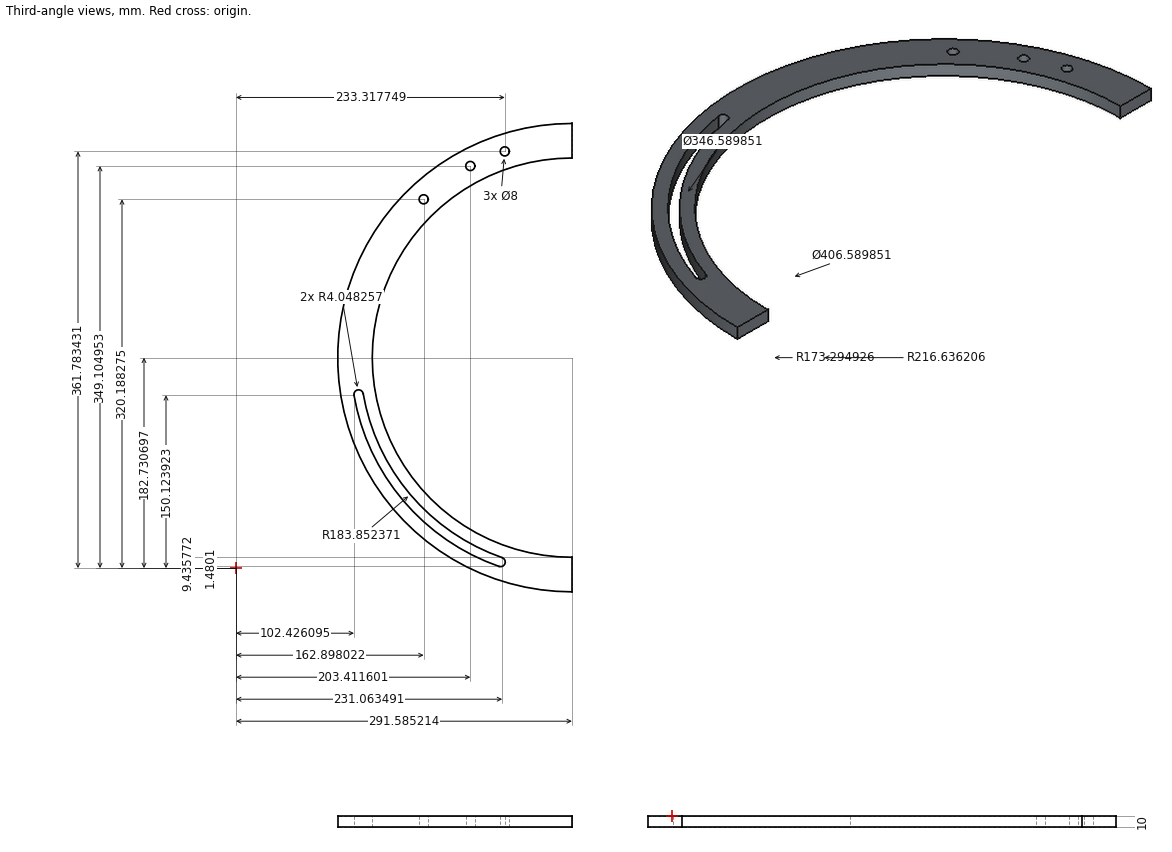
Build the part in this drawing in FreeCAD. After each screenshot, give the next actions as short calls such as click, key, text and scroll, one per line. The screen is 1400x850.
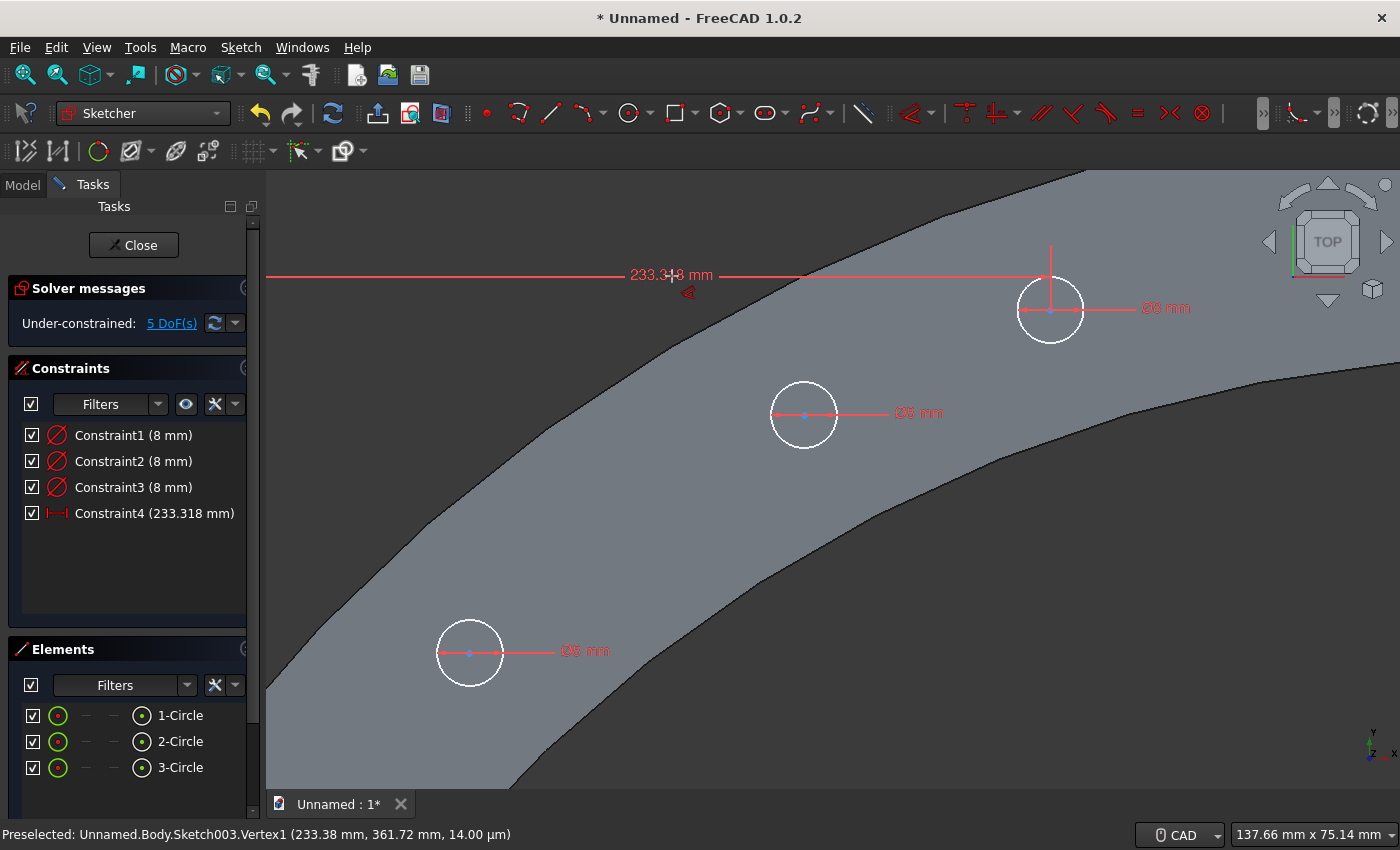
click(1051, 310)
click(1085, 536)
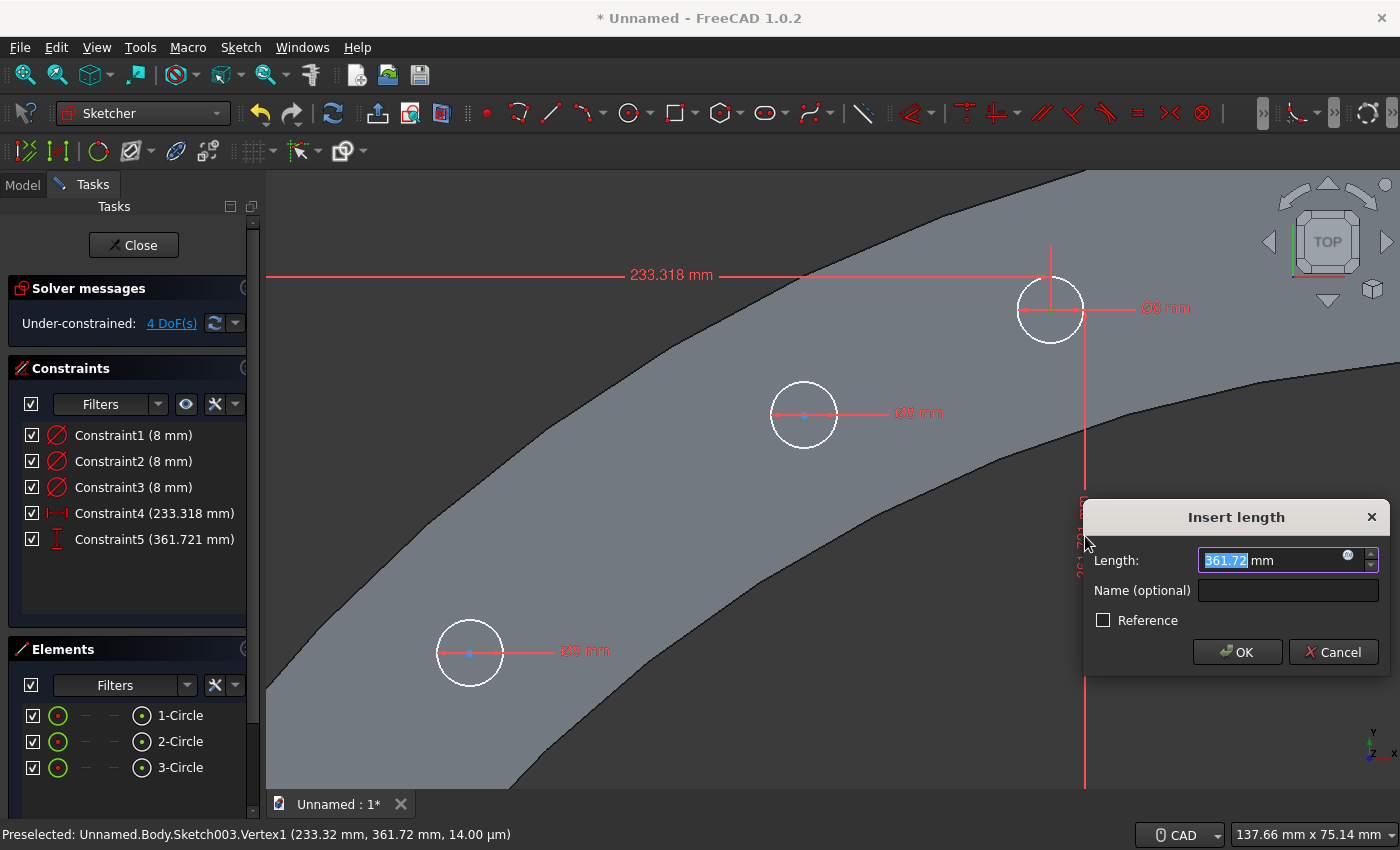
text(361.783431)
key(Return)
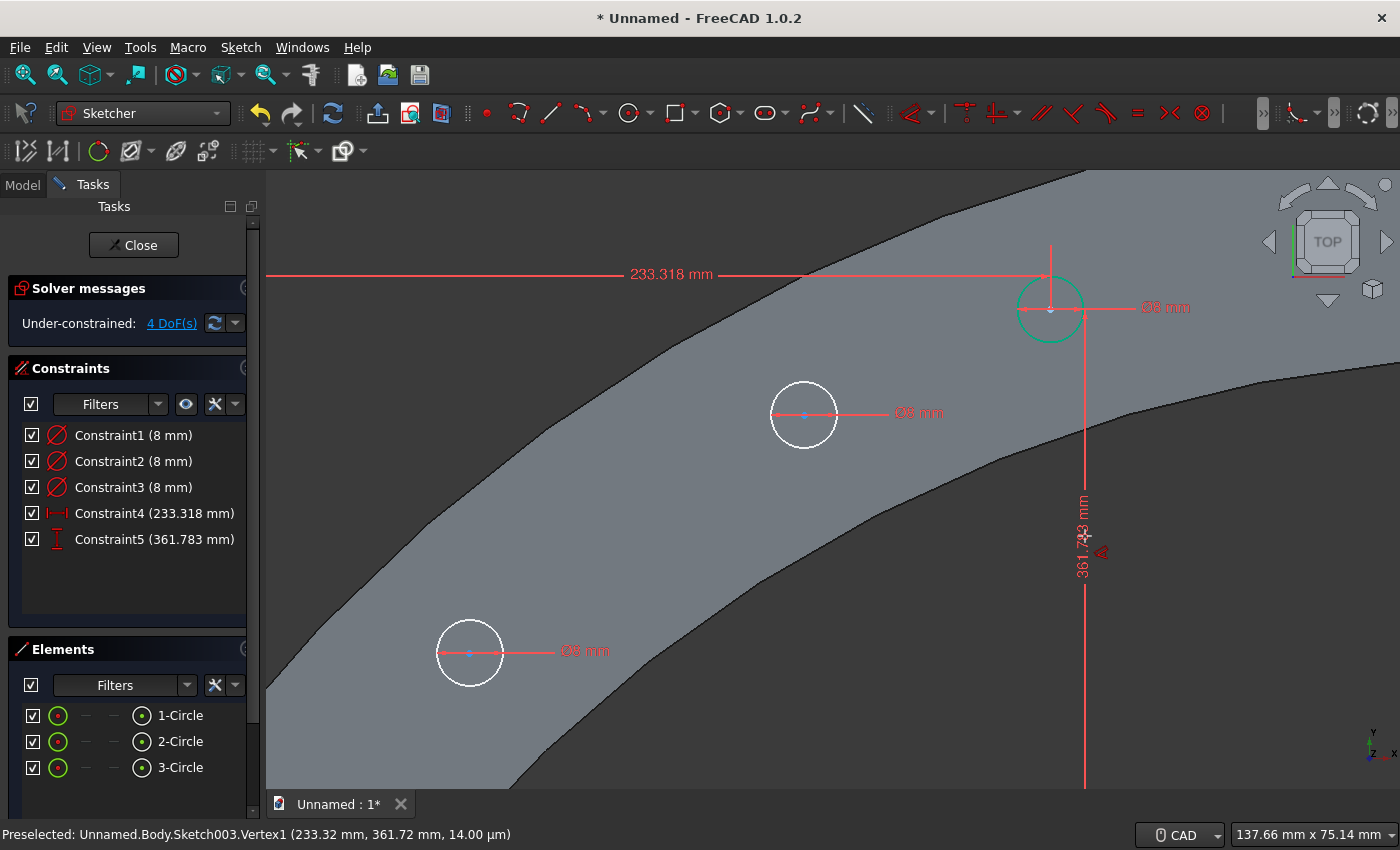
click(804, 415)
click(549, 381)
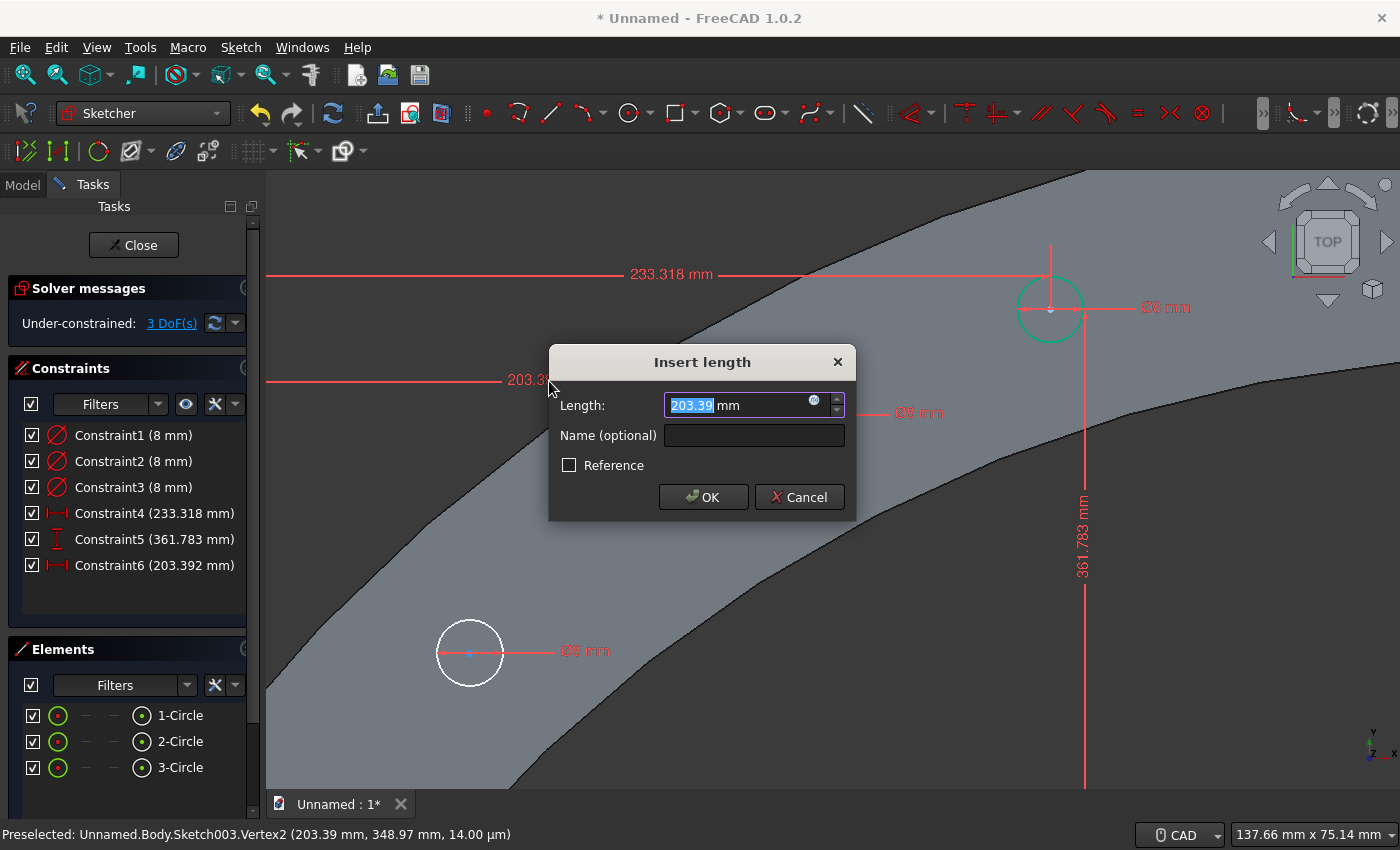
text(203.411601)
key(Return)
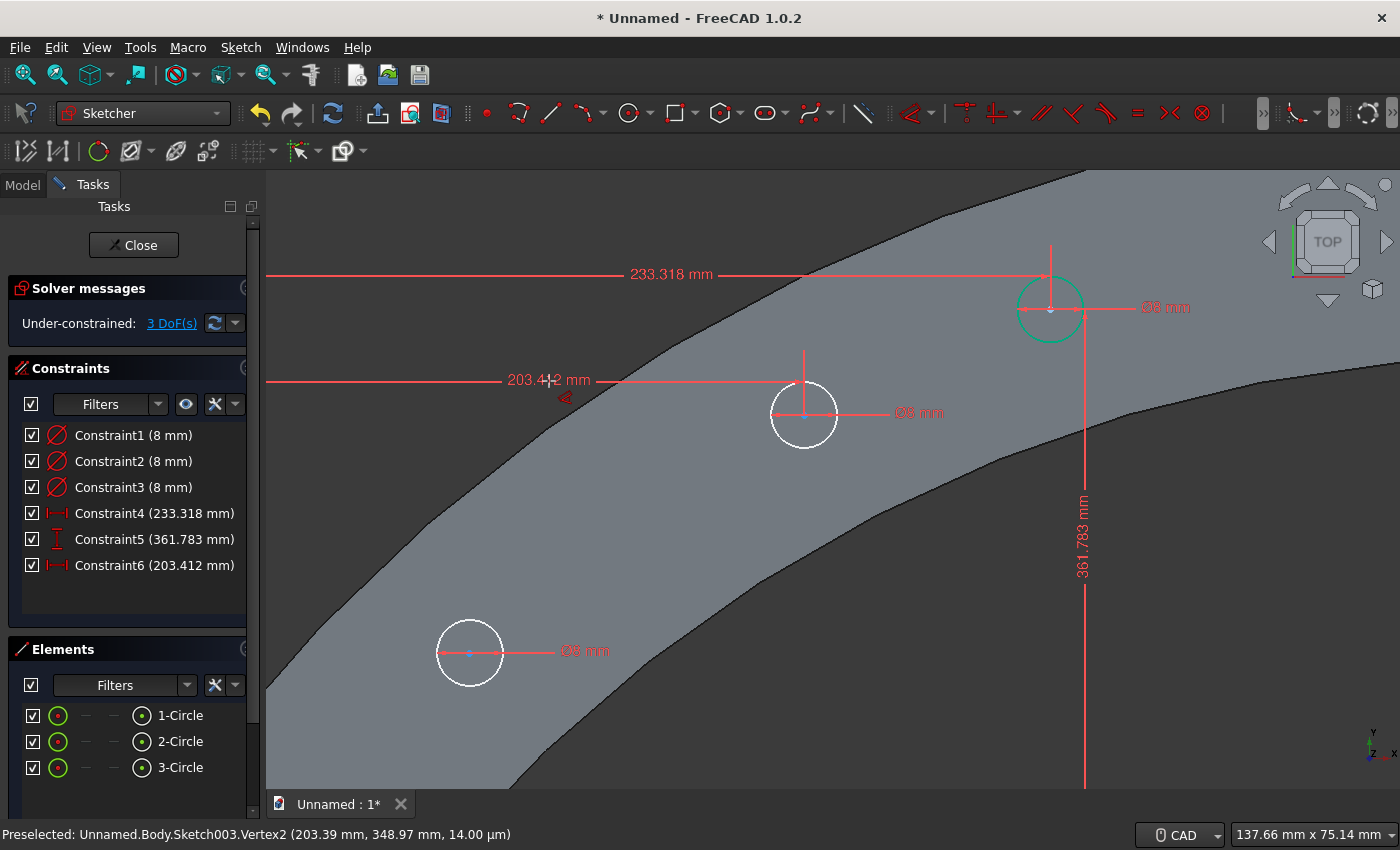
click(804, 415)
click(838, 588)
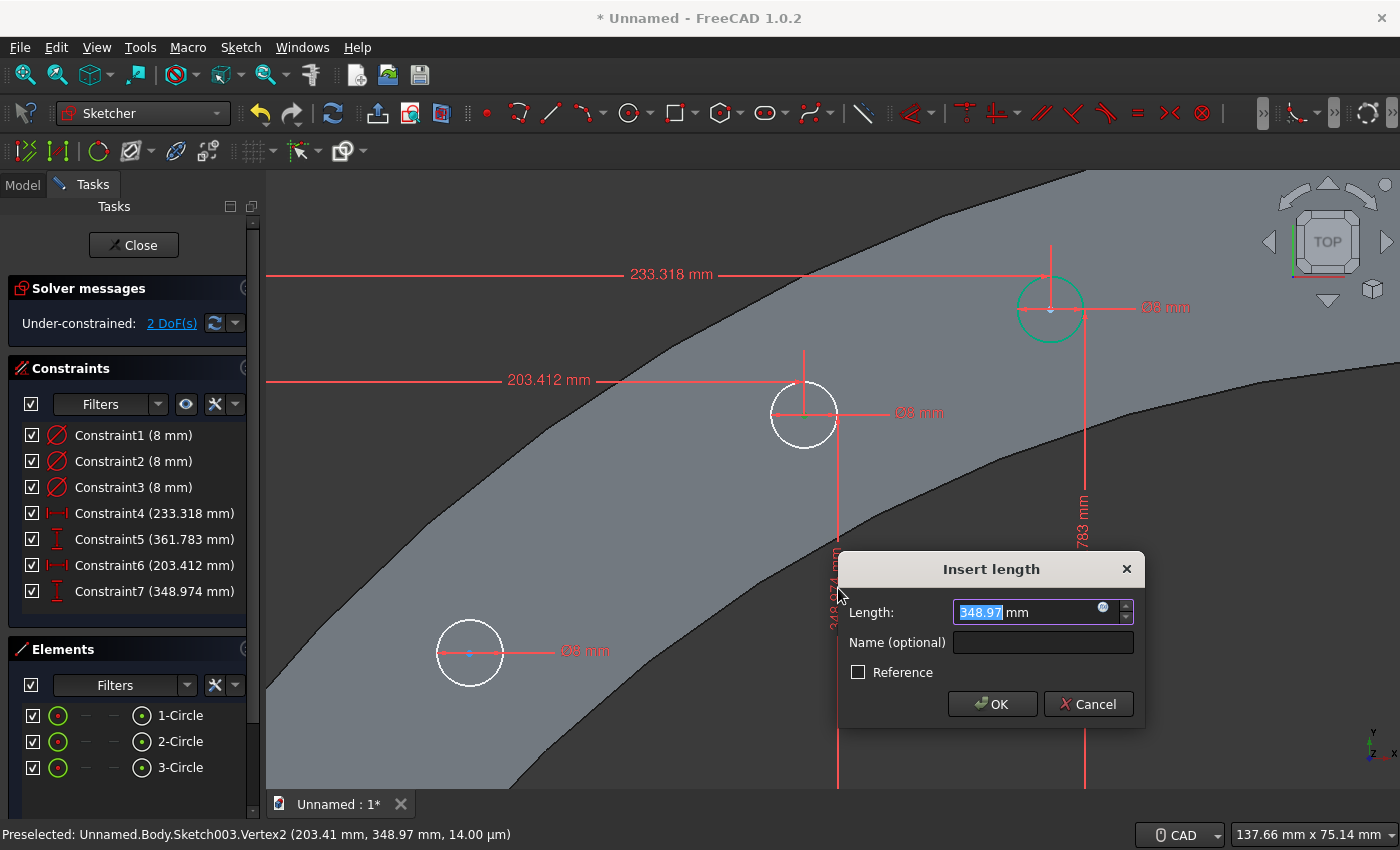
text(349.104953)
key(Return)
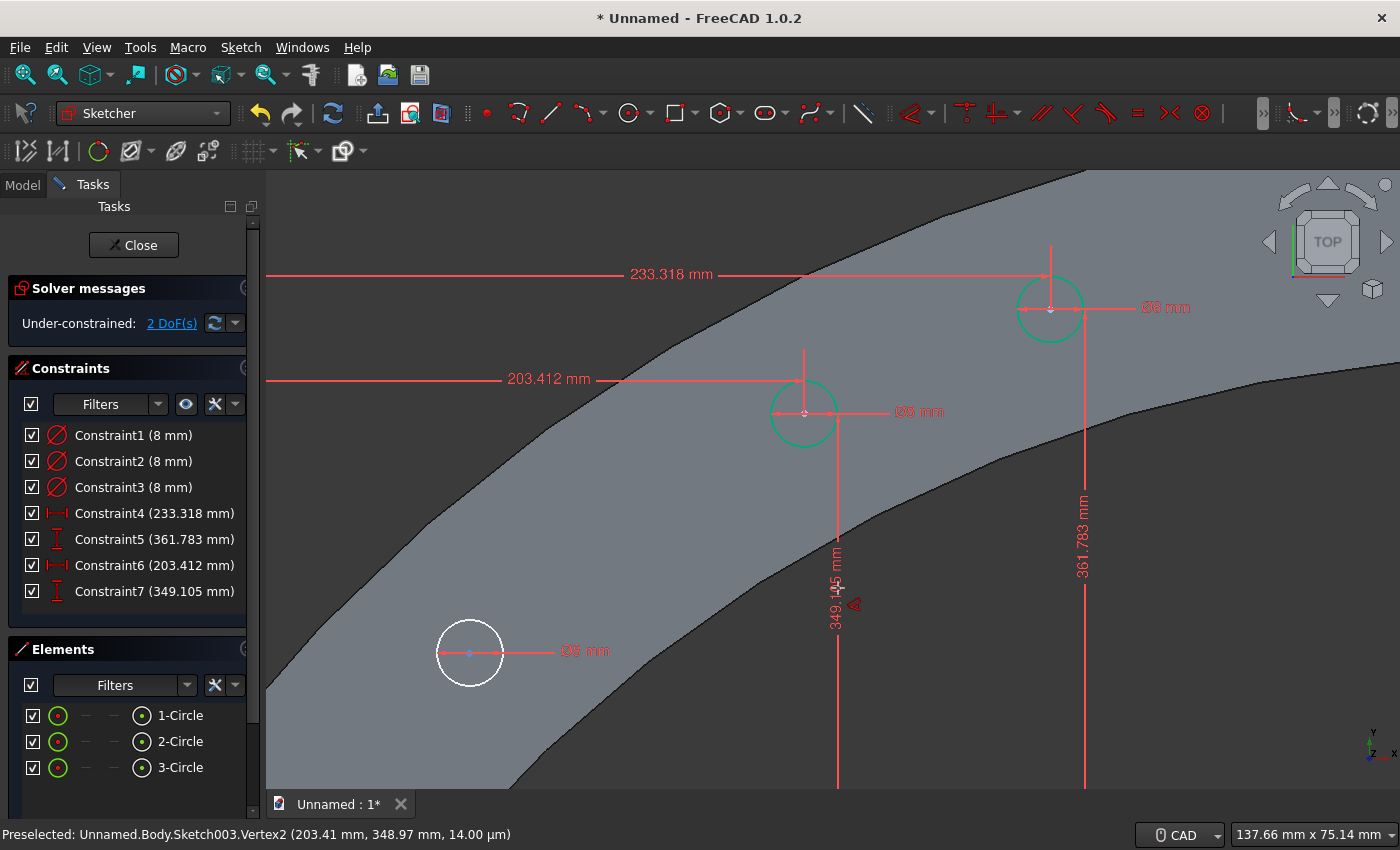
click(470, 653)
click(382, 619)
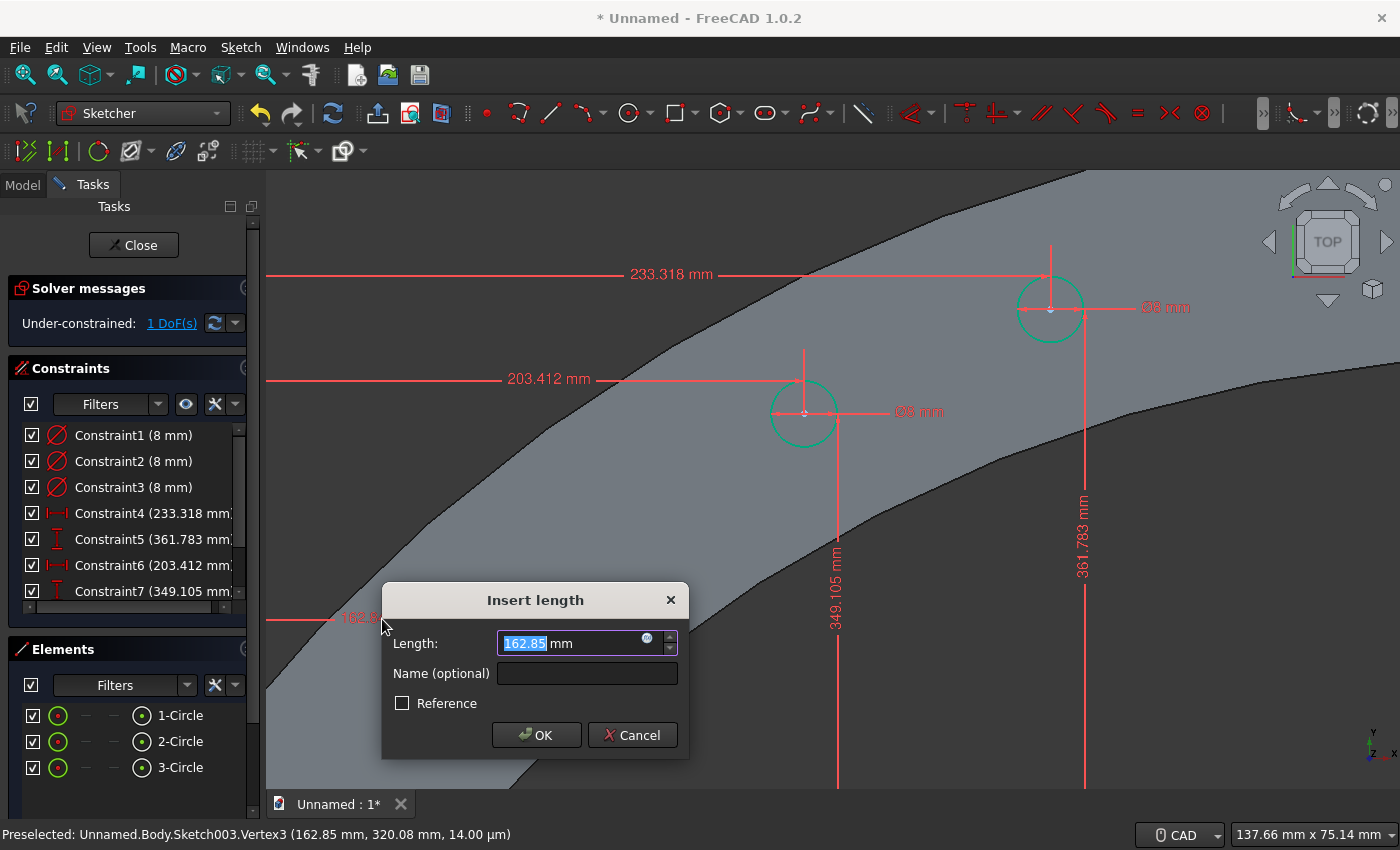
text(162.898022)
key(Return)